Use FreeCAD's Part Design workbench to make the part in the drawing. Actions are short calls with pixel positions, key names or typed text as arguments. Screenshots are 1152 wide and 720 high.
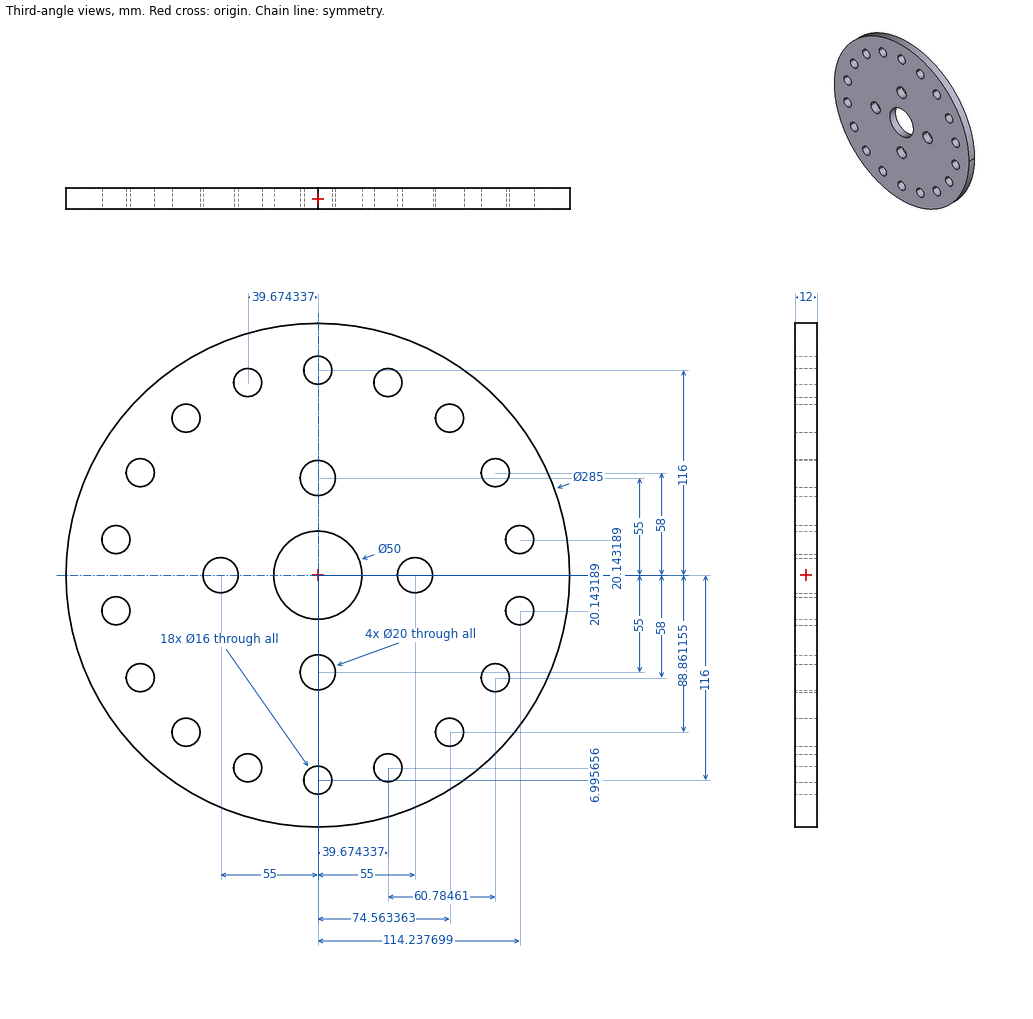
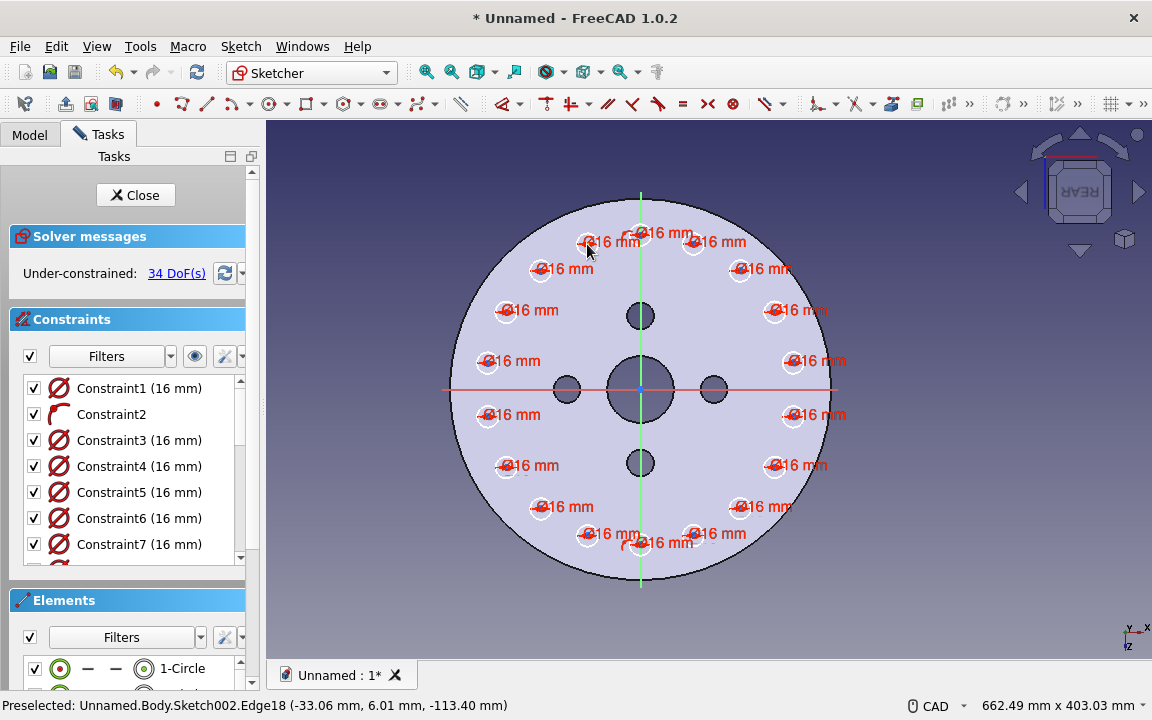
click(793, 363)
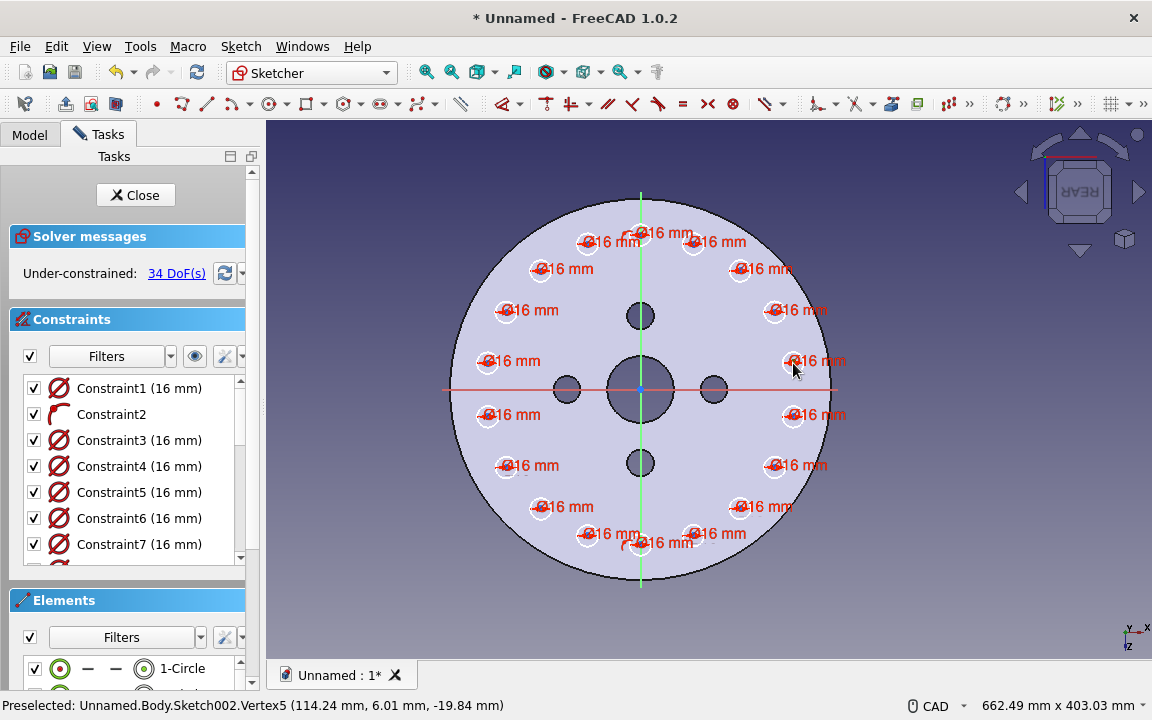
click(793, 417)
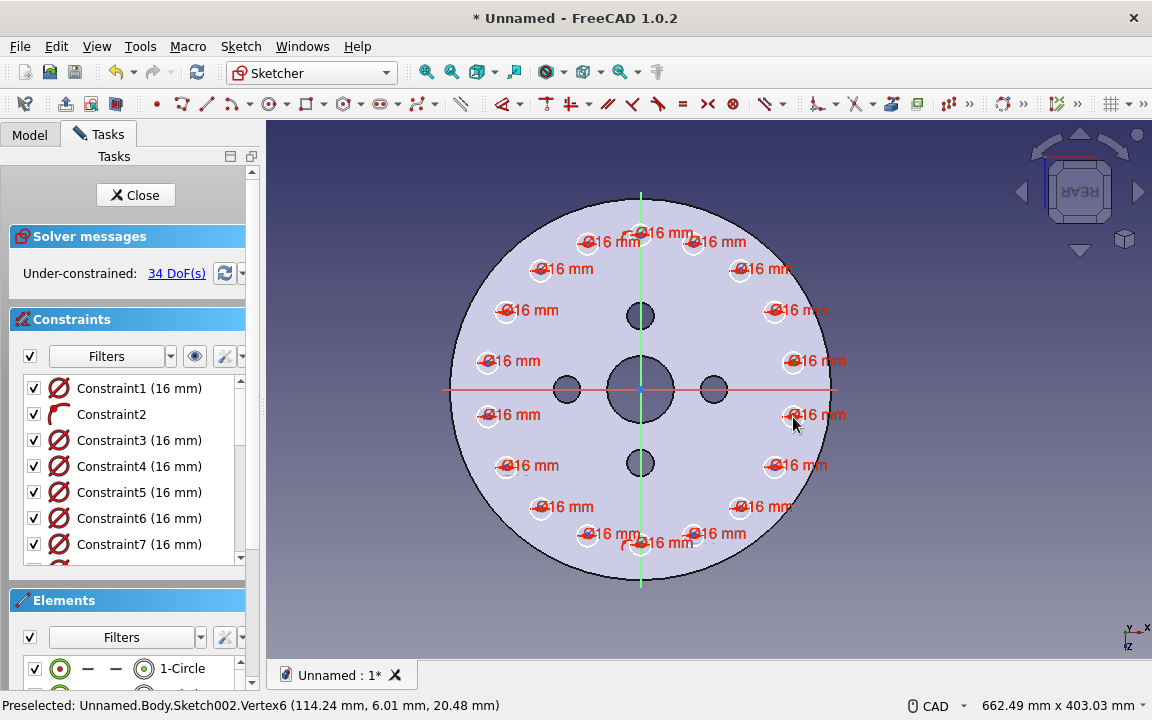
click(588, 104)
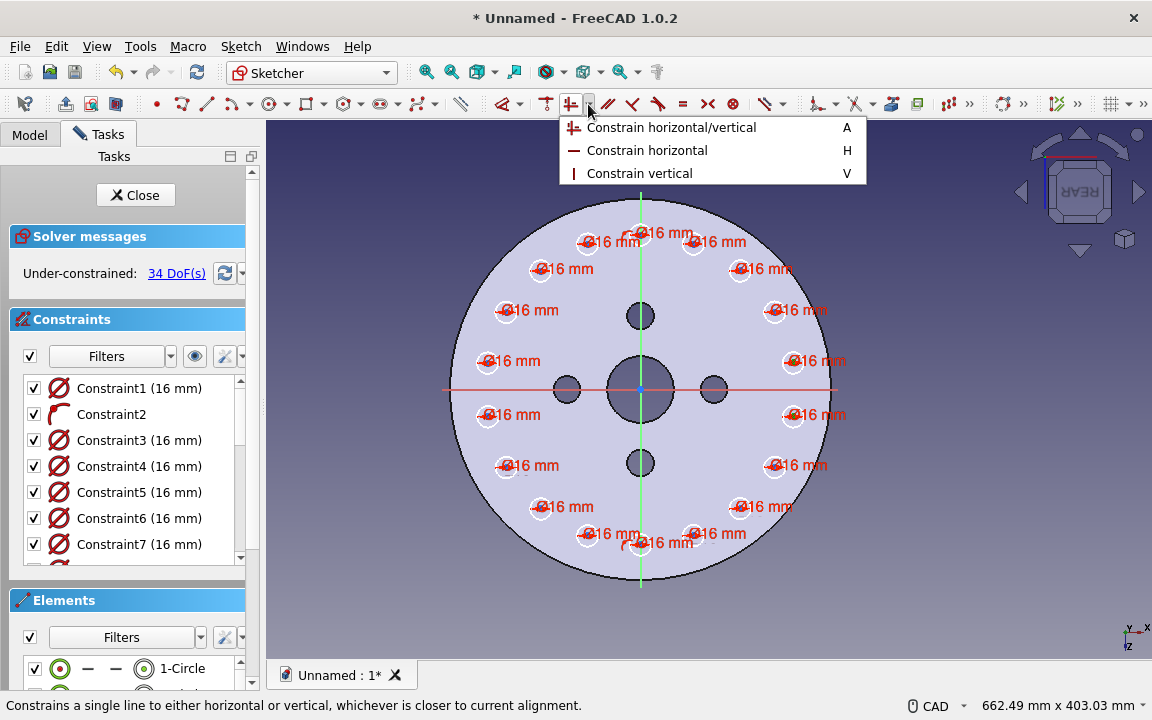
click(713, 174)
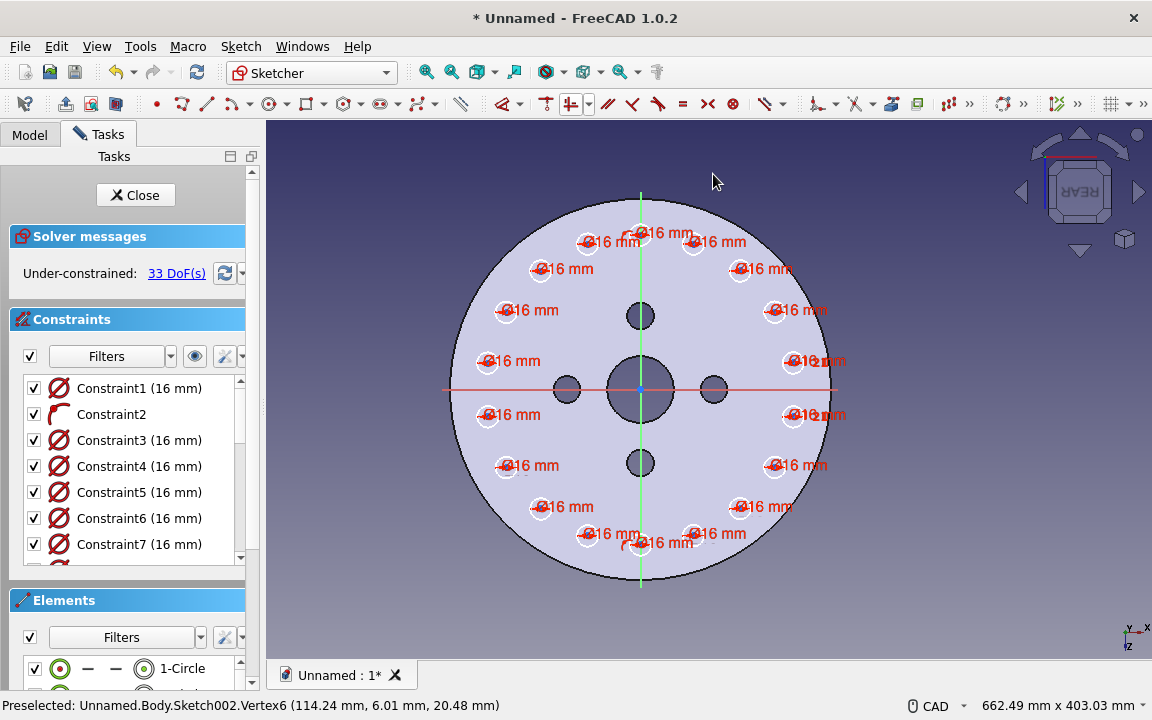
click(775, 312)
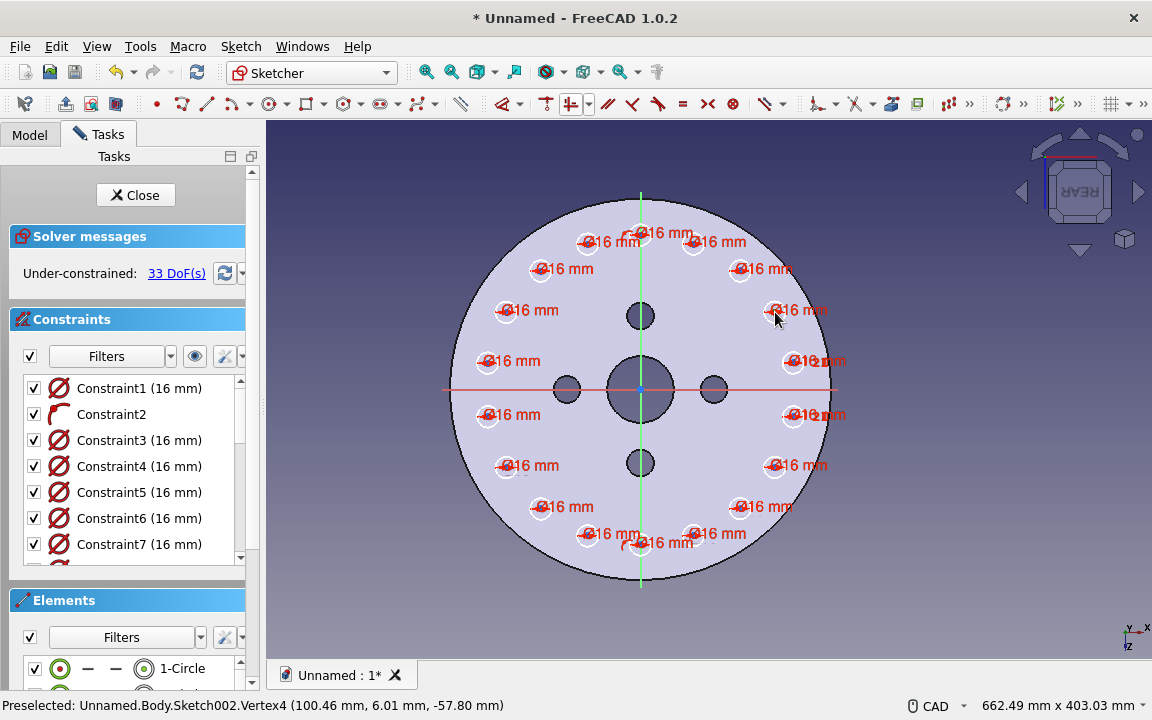
click(775, 467)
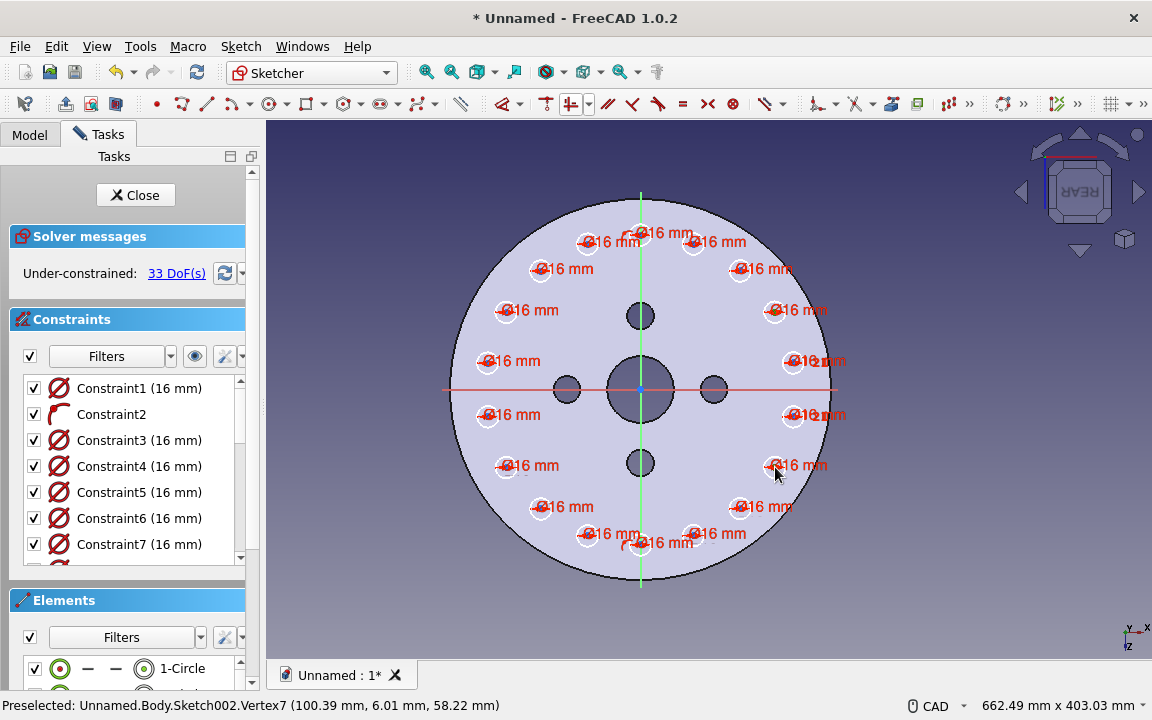
key(v)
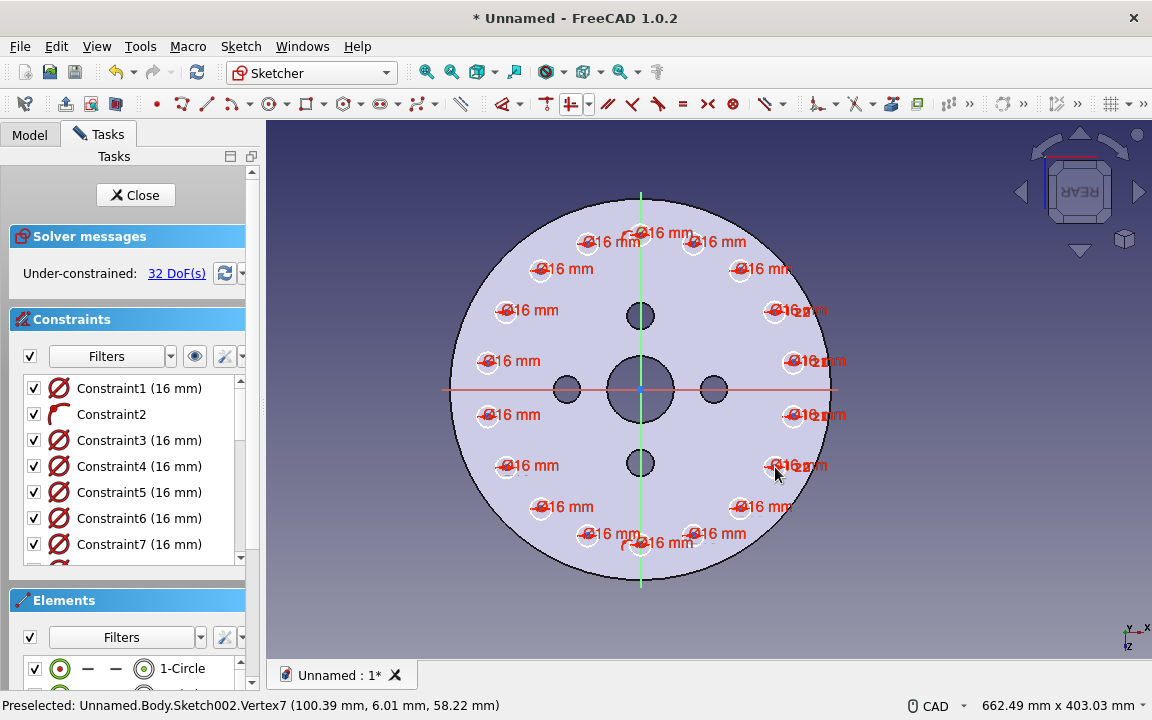
click(740, 271)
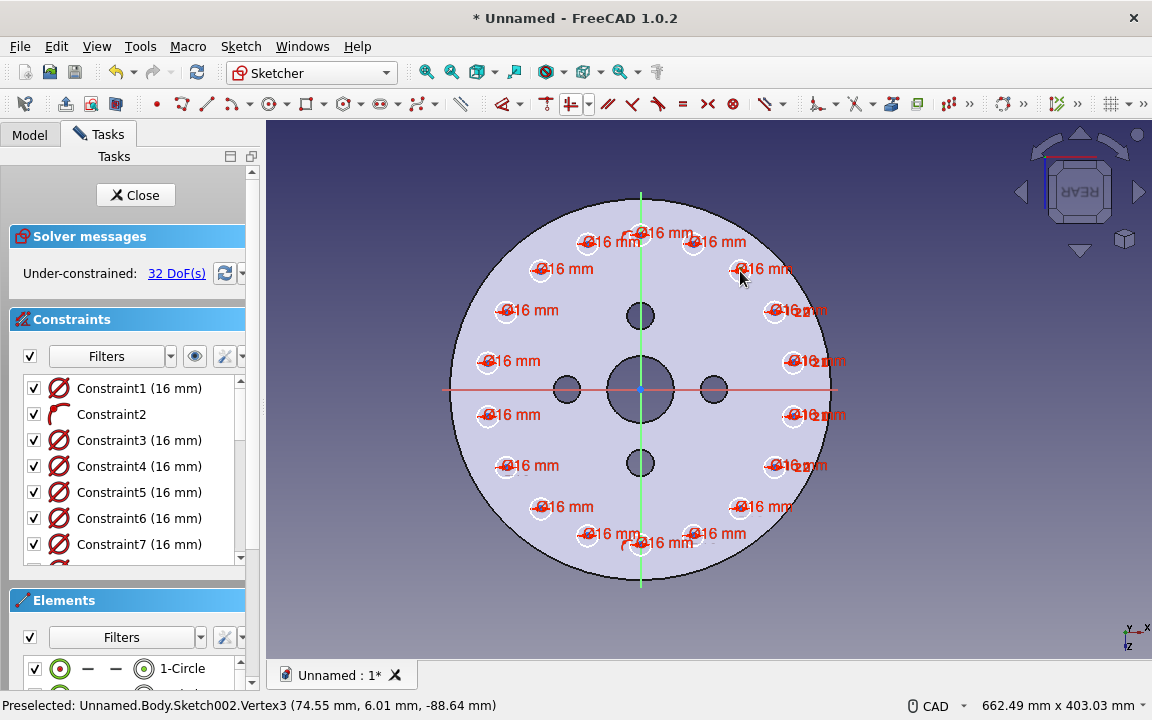
click(740, 509)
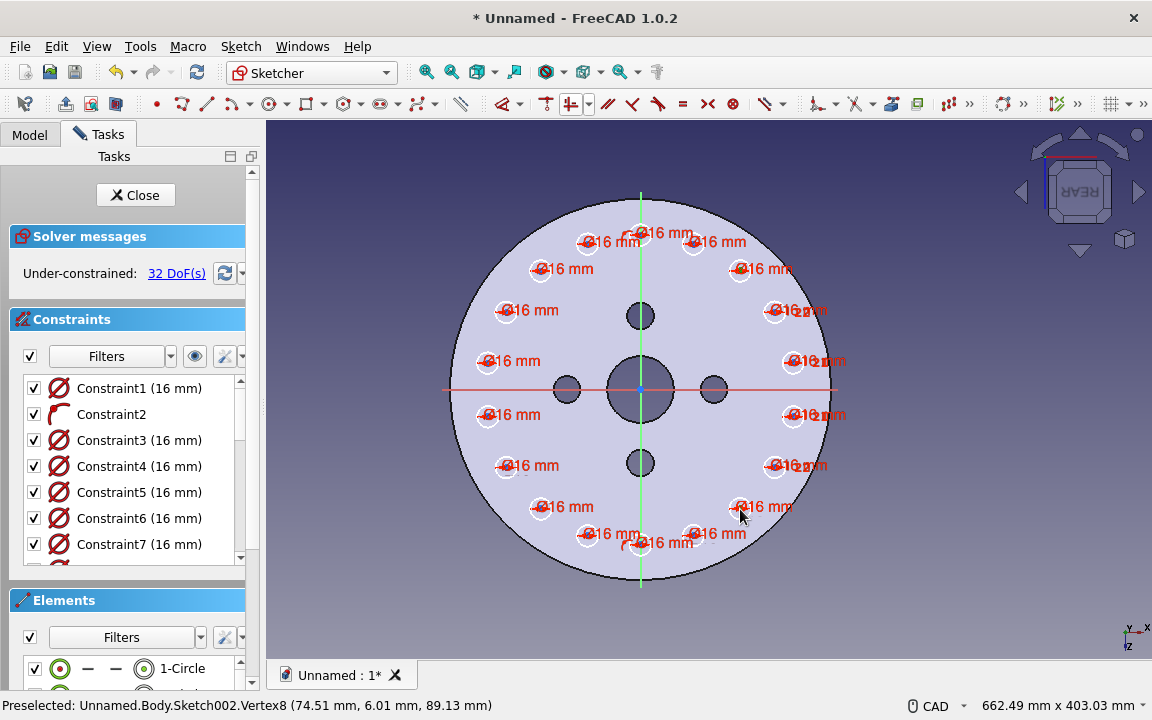
key(v)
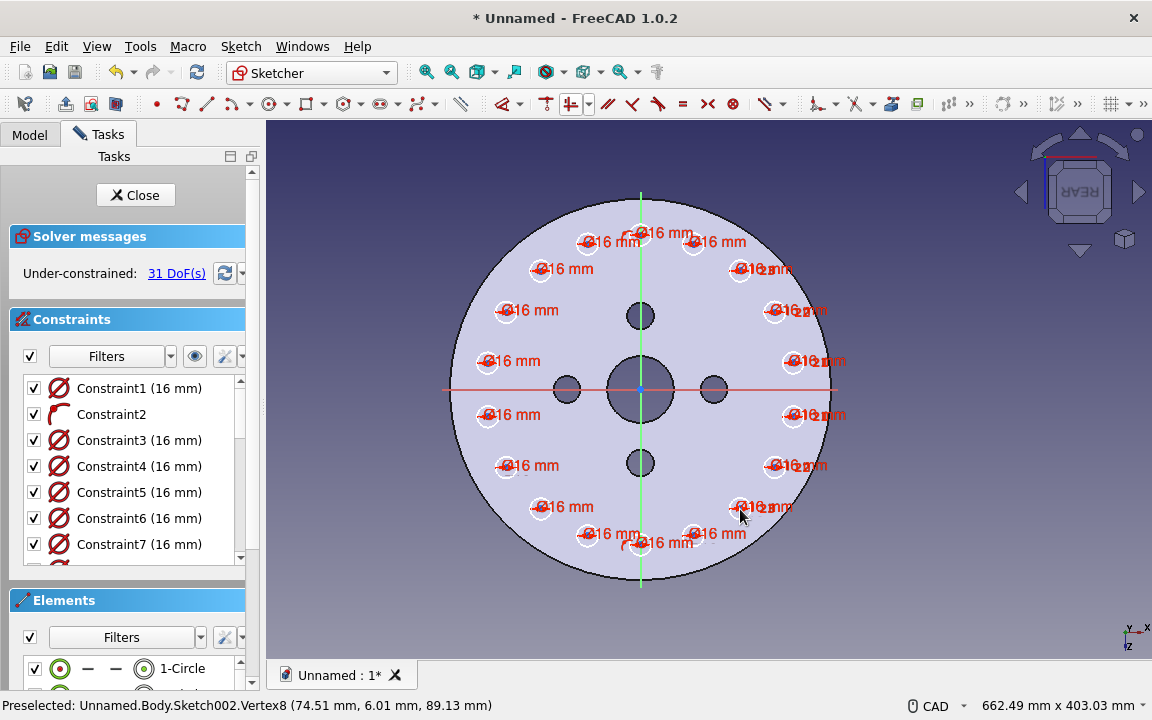
click(693, 536)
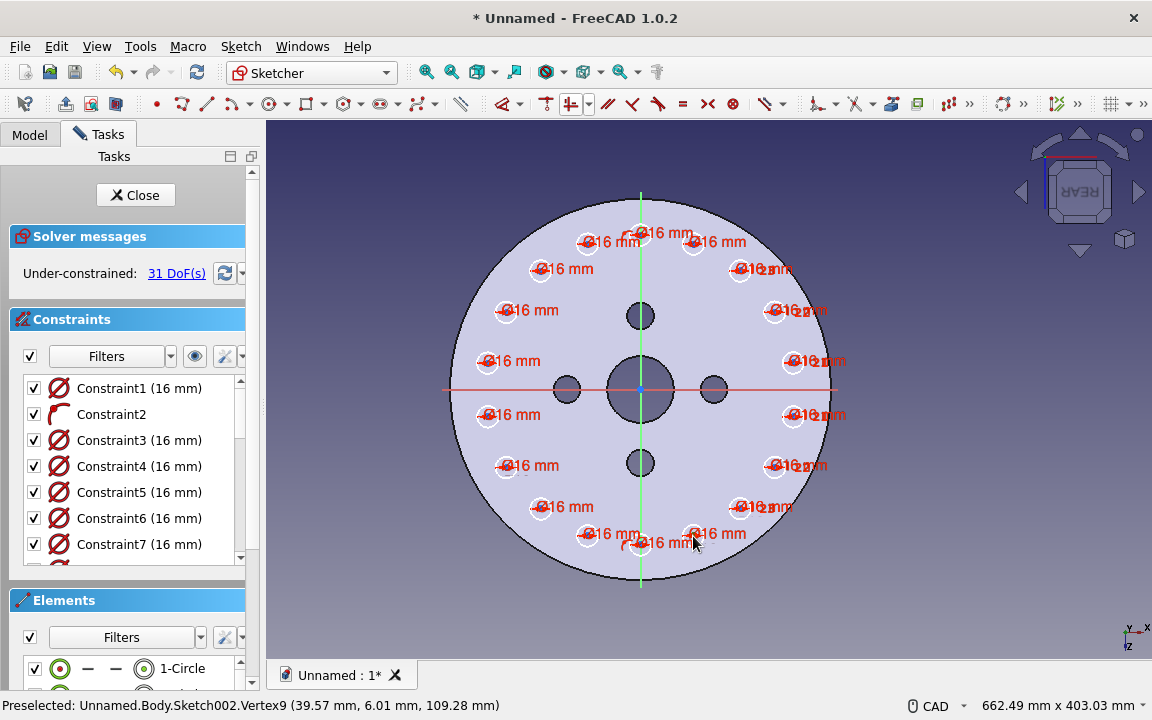
click(588, 536)